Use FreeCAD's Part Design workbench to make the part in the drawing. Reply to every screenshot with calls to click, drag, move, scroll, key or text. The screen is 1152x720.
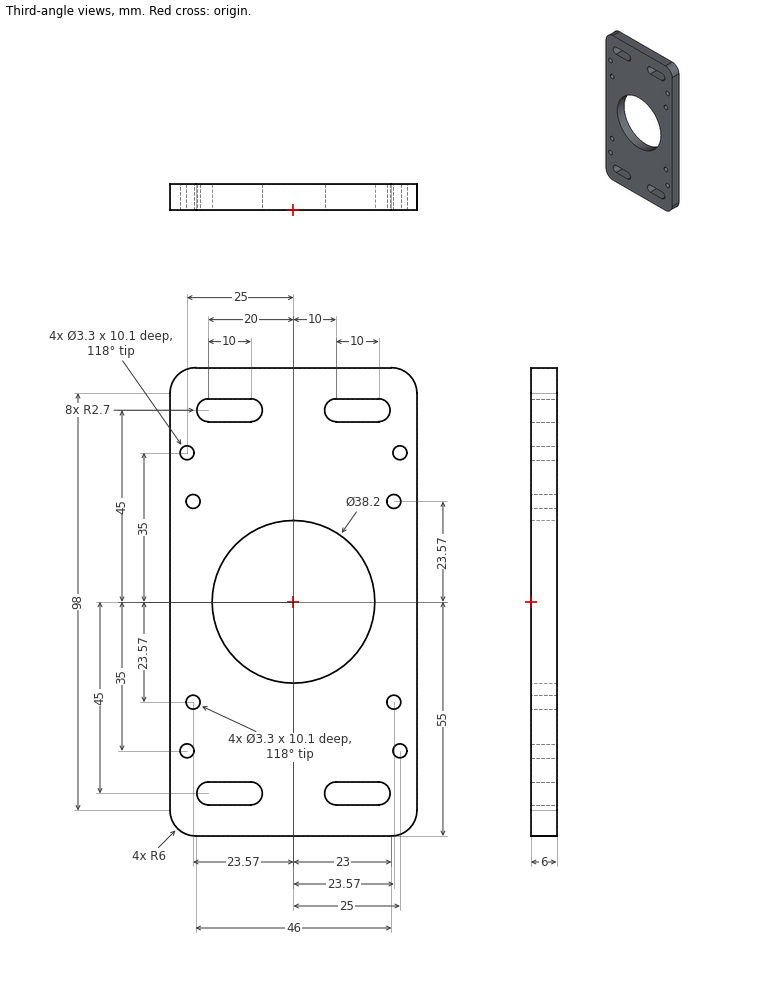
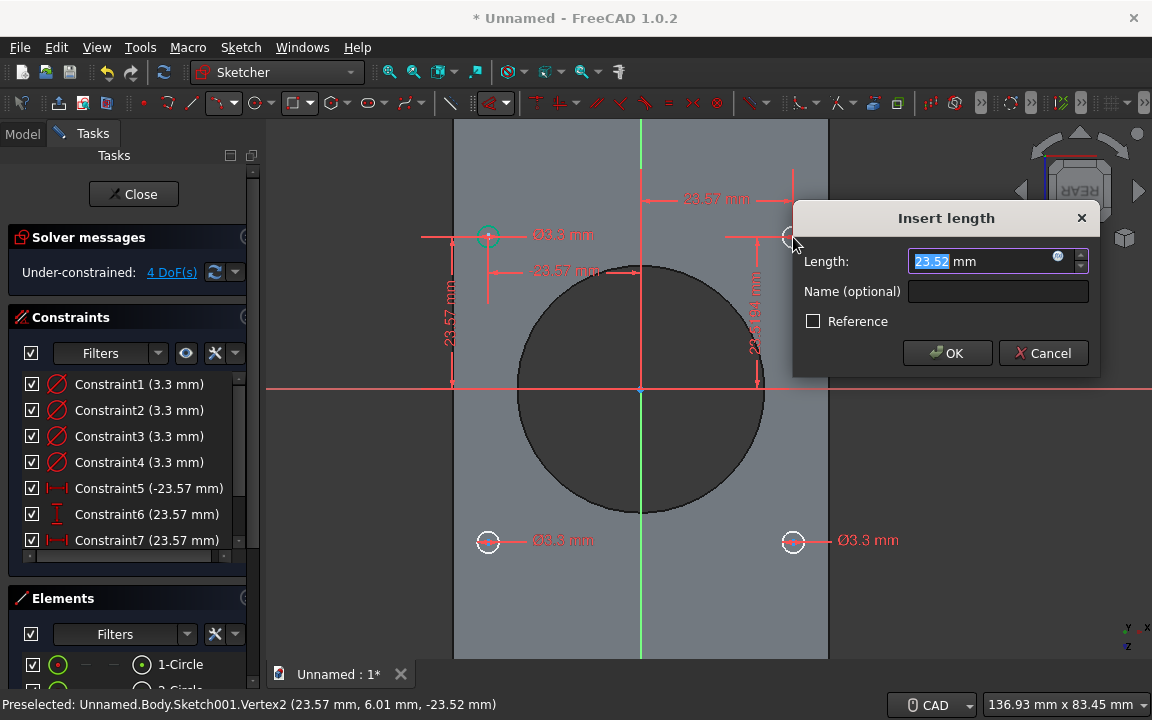
text(23.57)
key(Return)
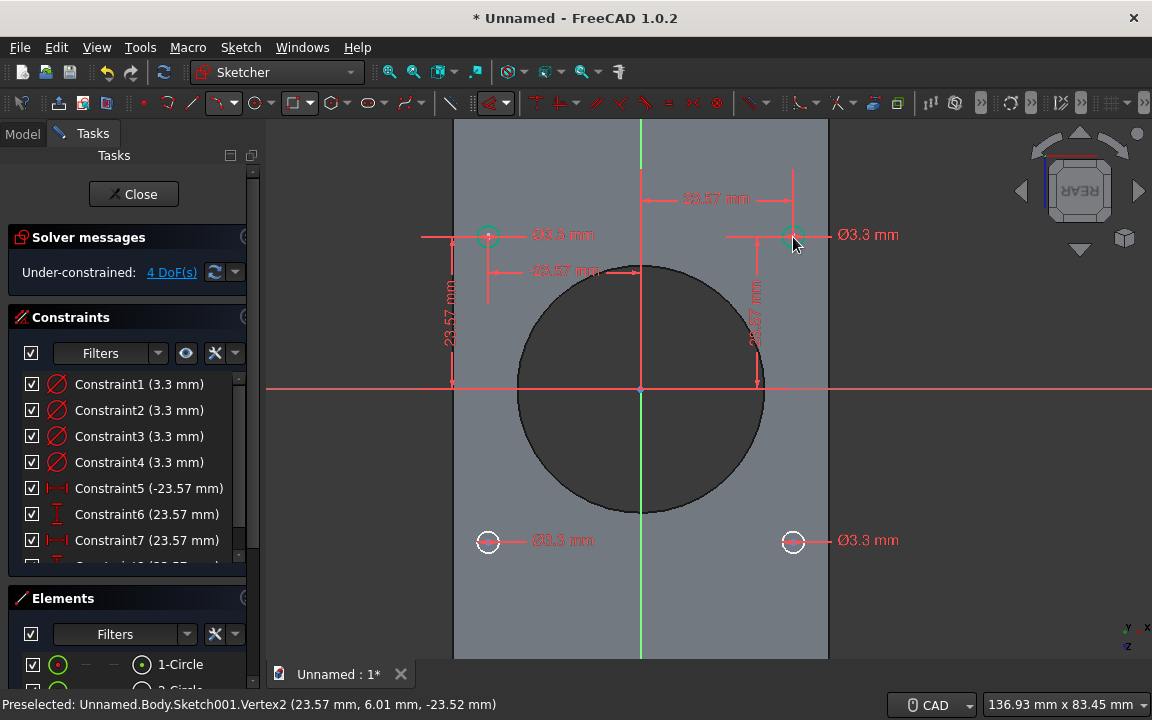
click(793, 542)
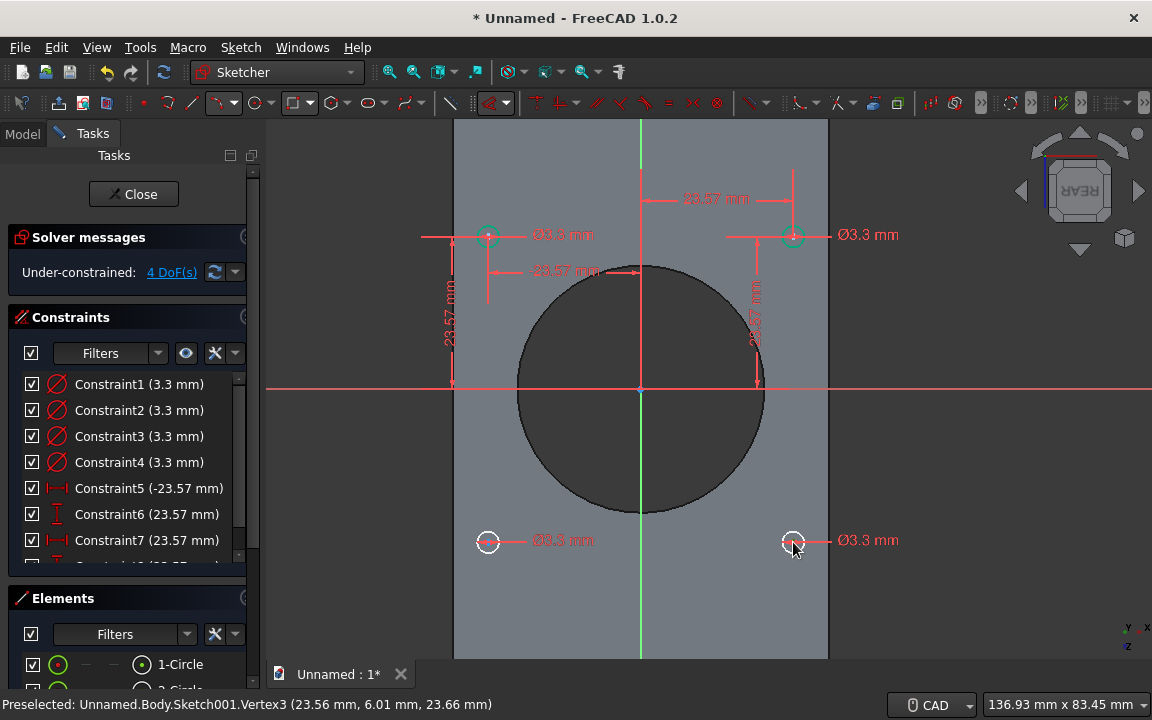
click(508, 104)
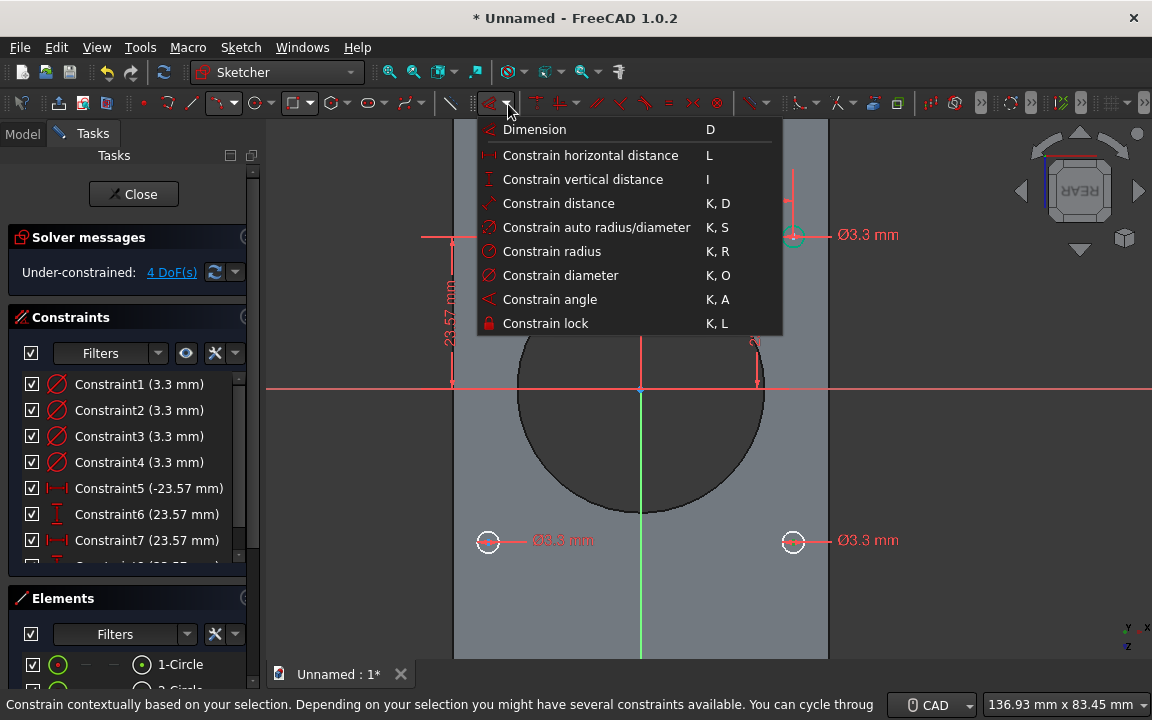
click(630, 155)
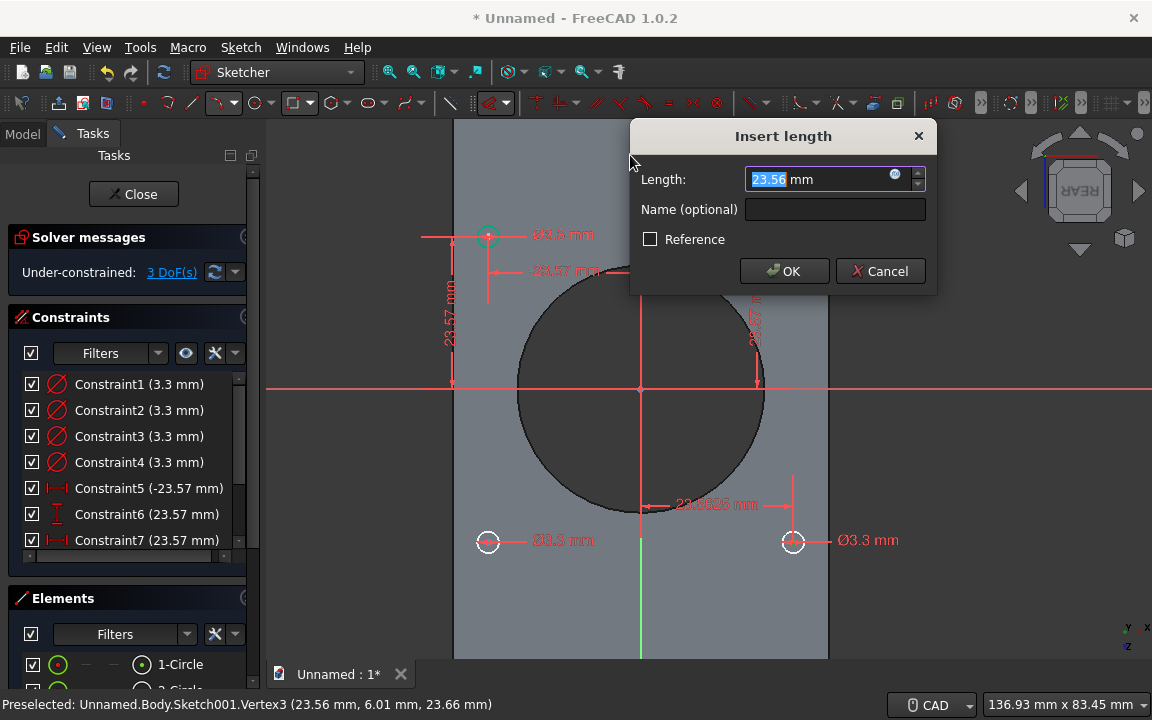
text(23.57)
key(Return)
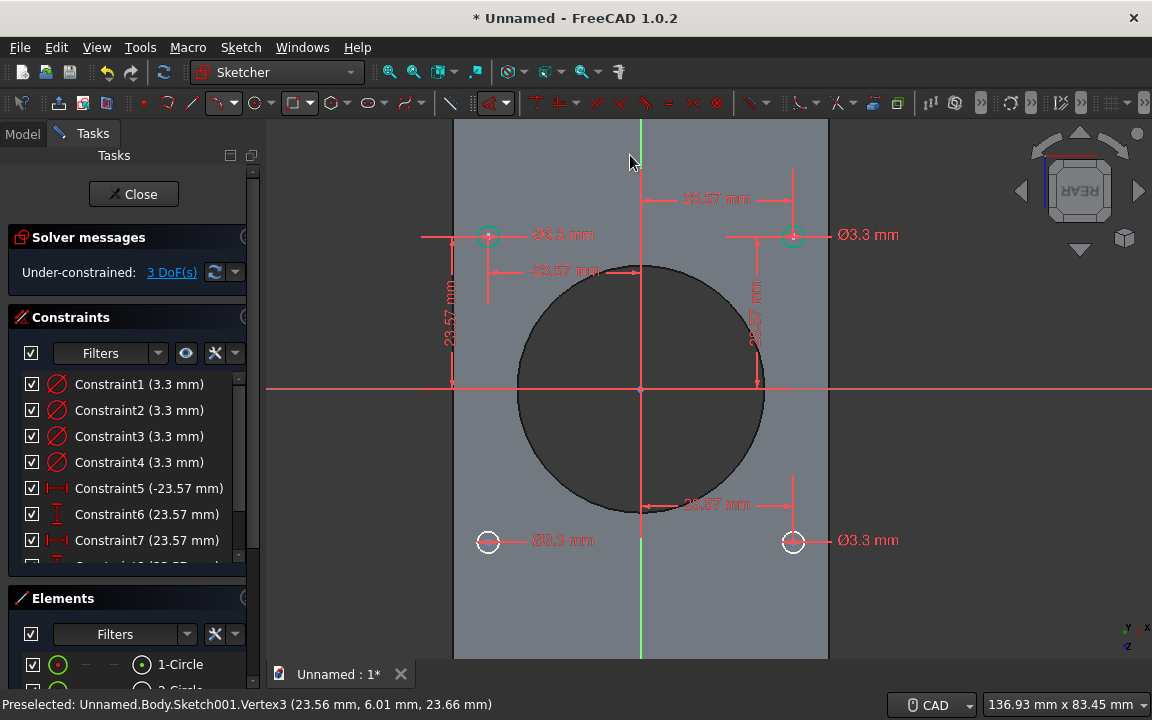
click(793, 542)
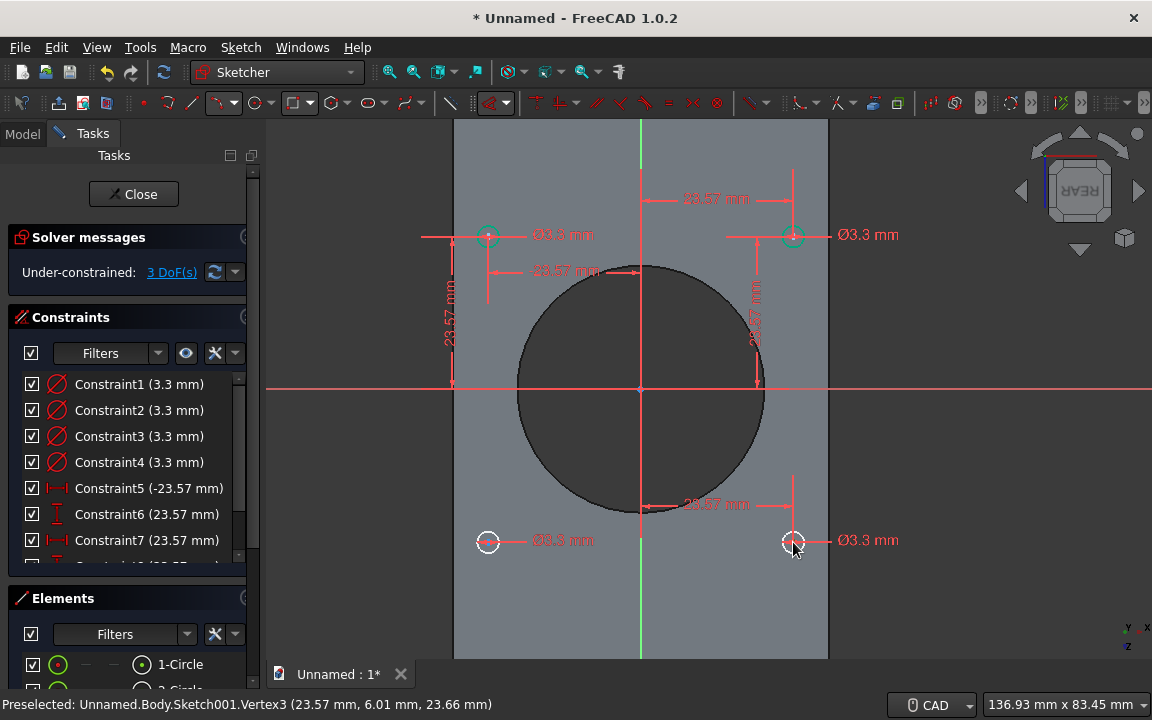
key(i)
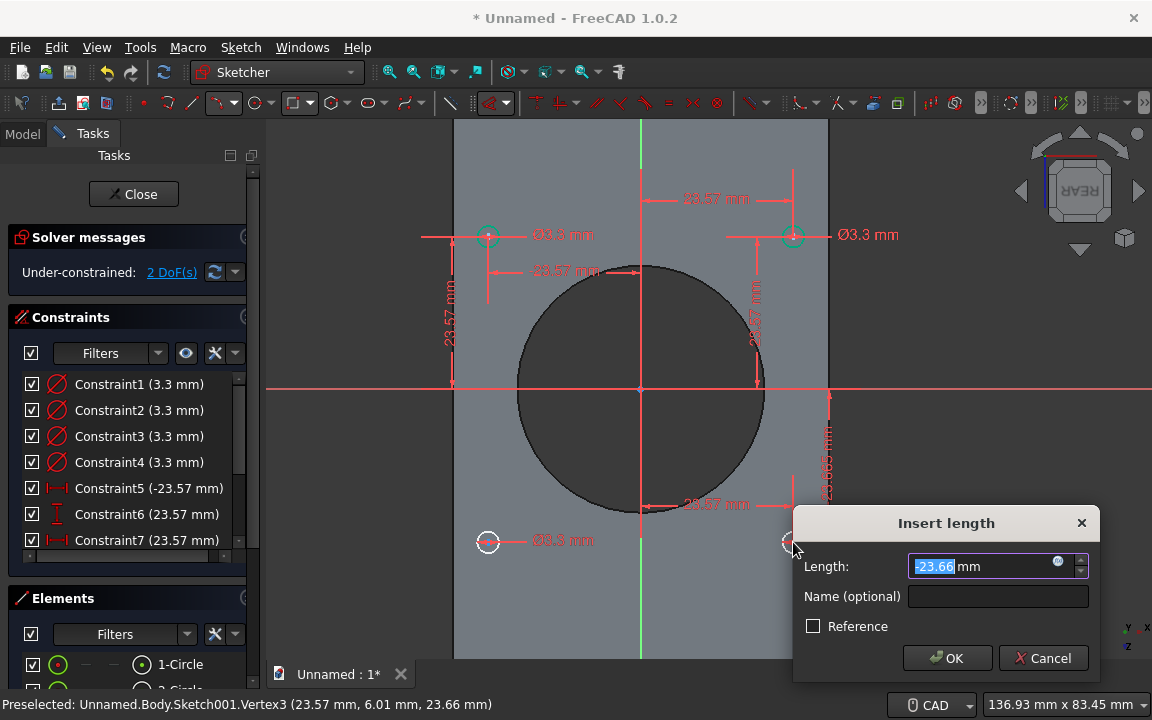
text(-23.57)
key(Return)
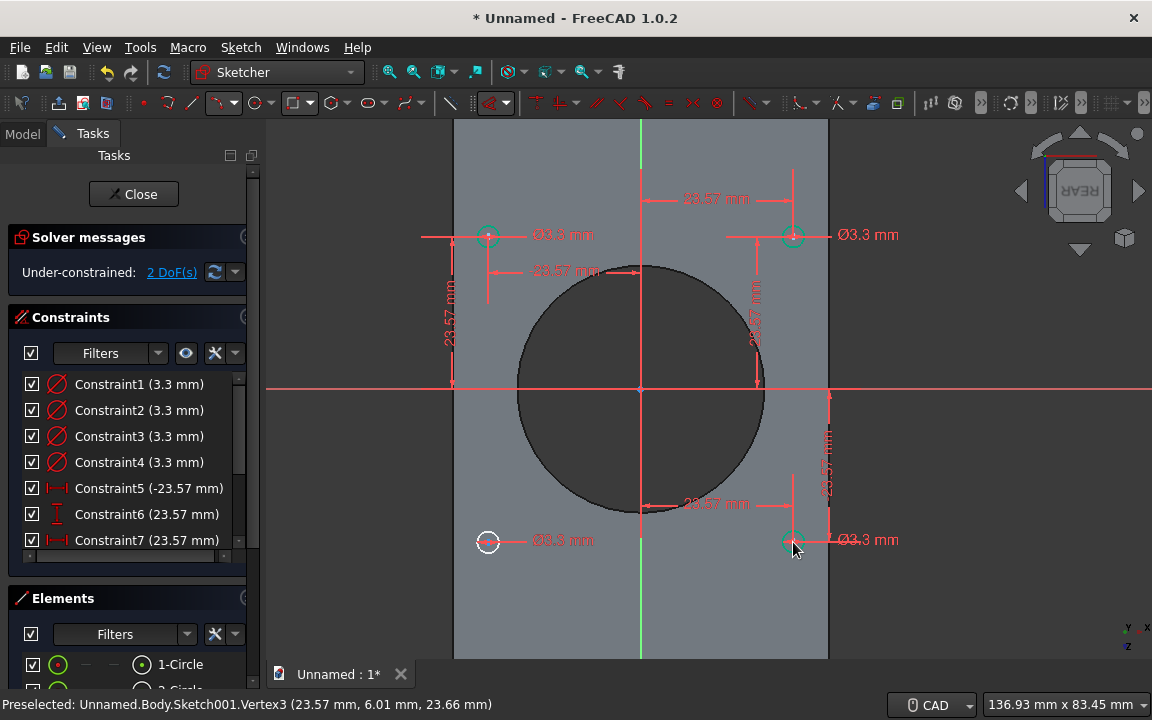
click(488, 542)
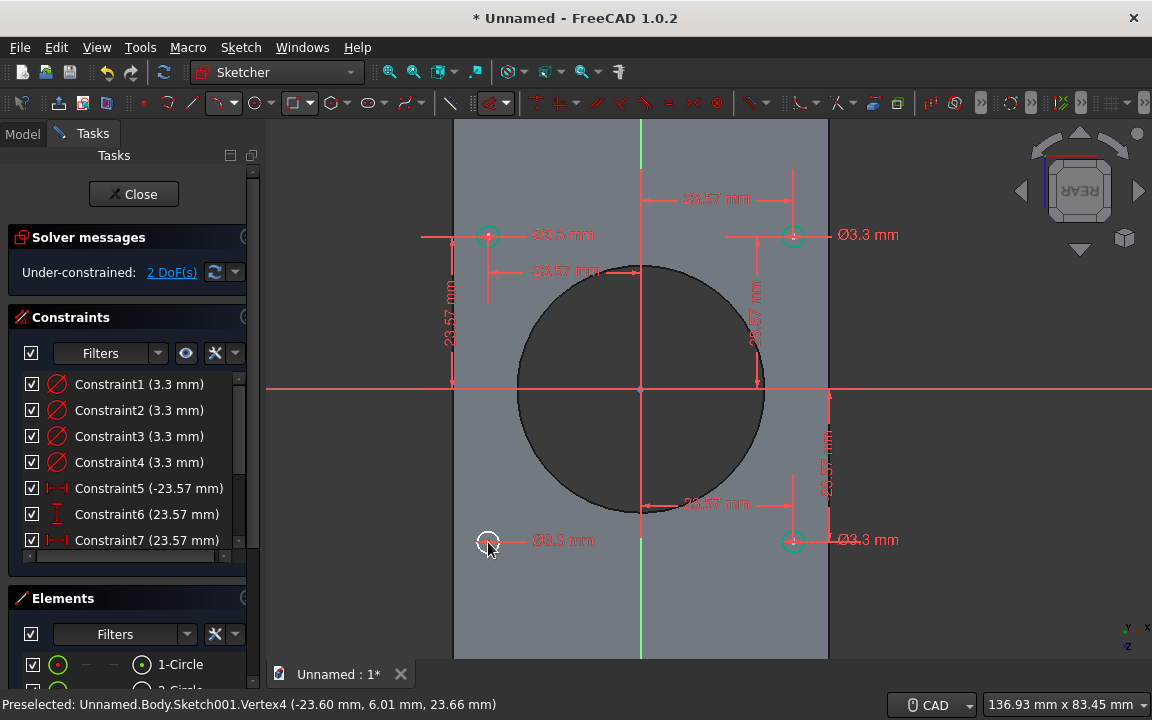
click(508, 104)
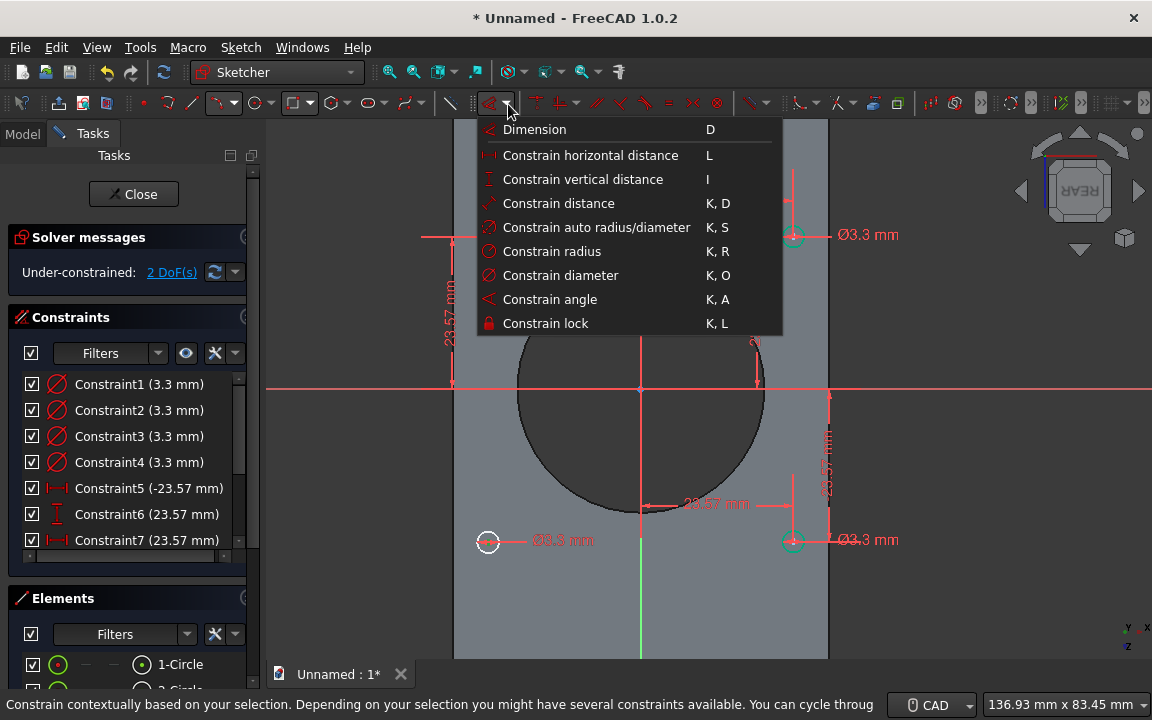
click(630, 155)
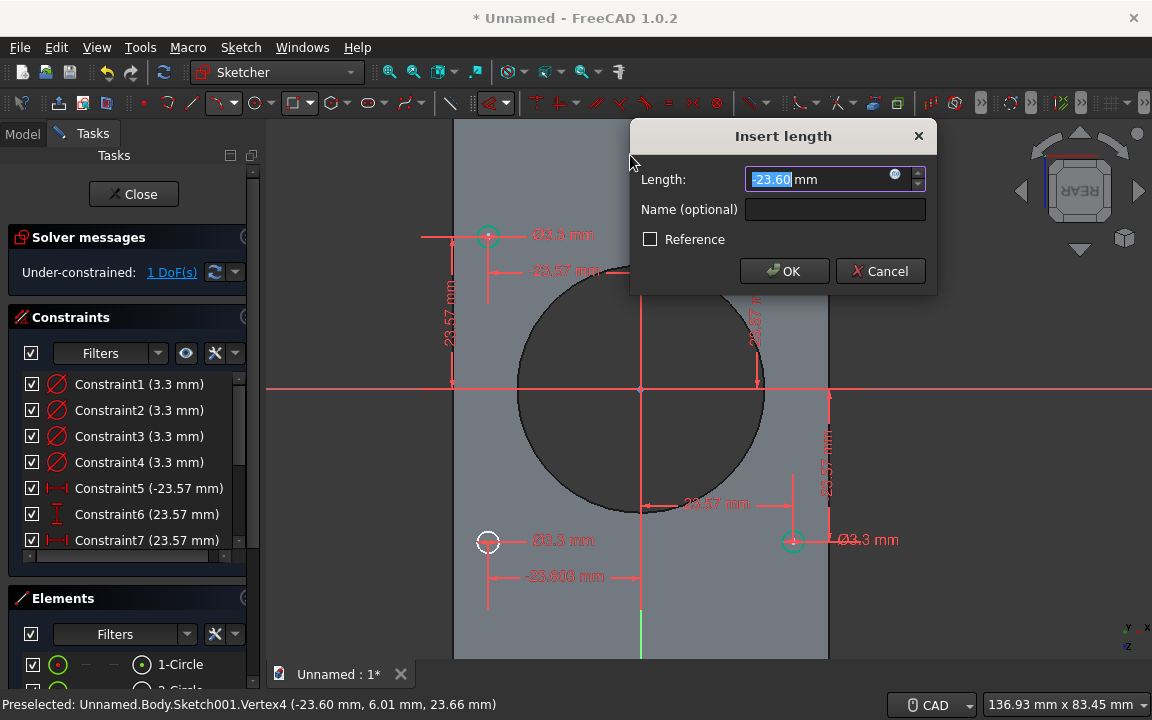
text(-23.57)
key(Return)